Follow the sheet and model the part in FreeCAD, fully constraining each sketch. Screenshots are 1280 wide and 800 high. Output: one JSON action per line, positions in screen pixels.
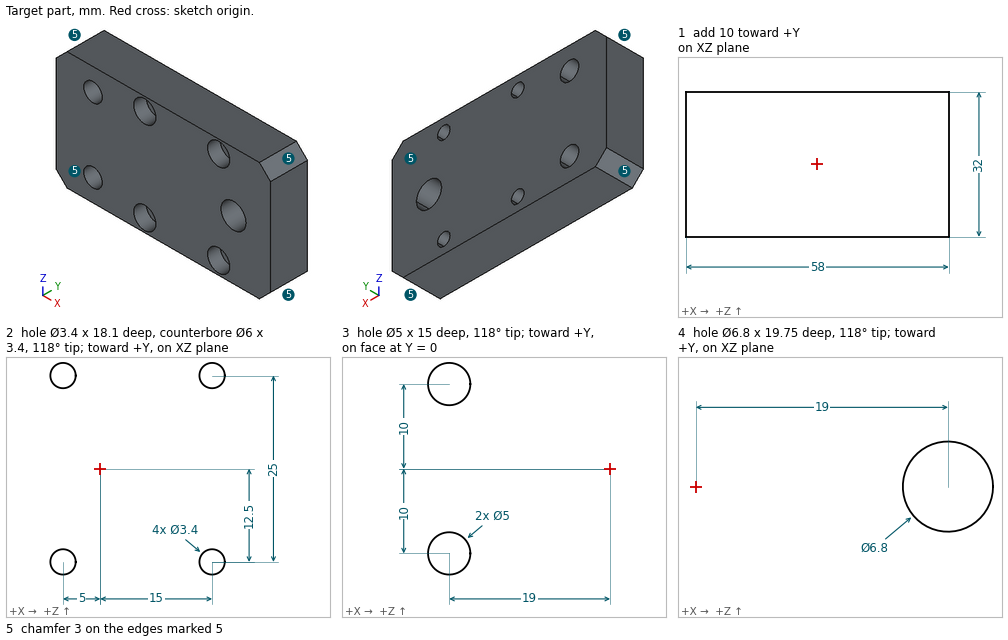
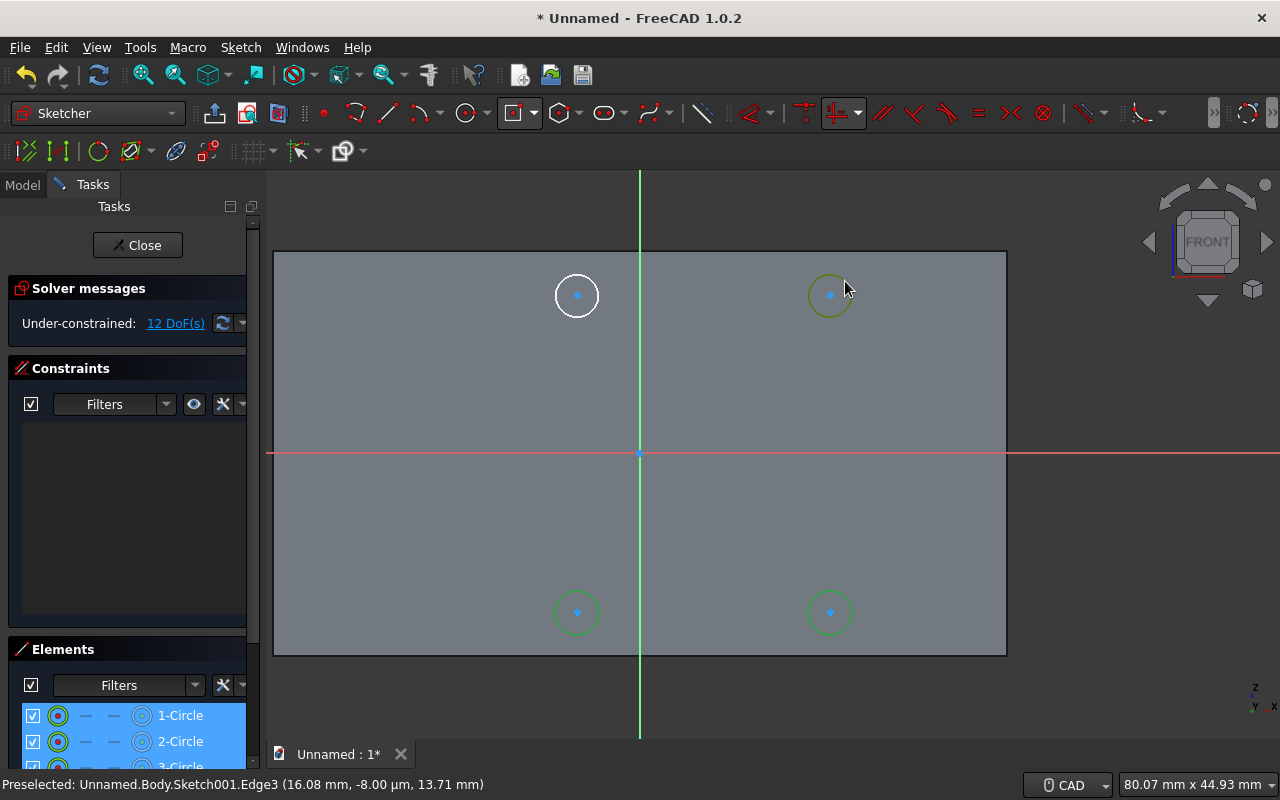
{"action": "left_click", "coordinate": [592, 281]}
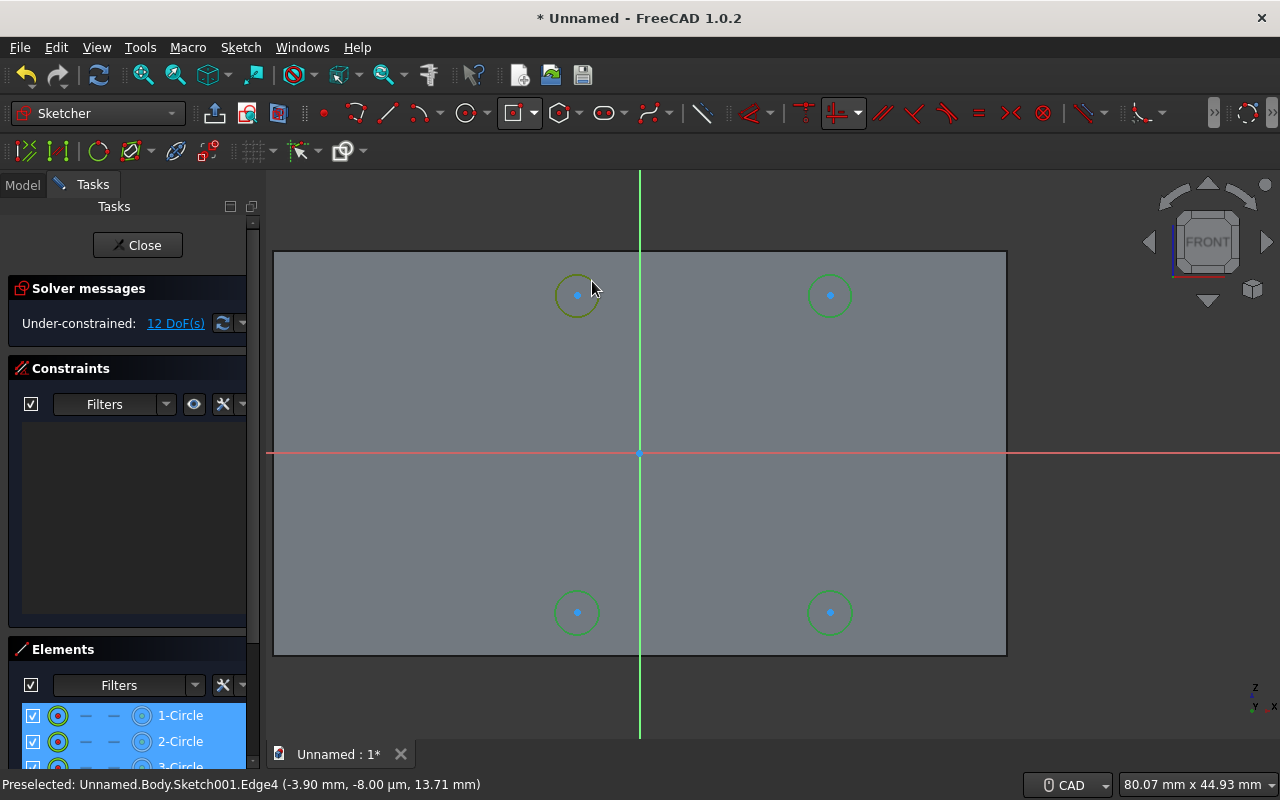
{"action": "left_click", "coordinate": [980, 114]}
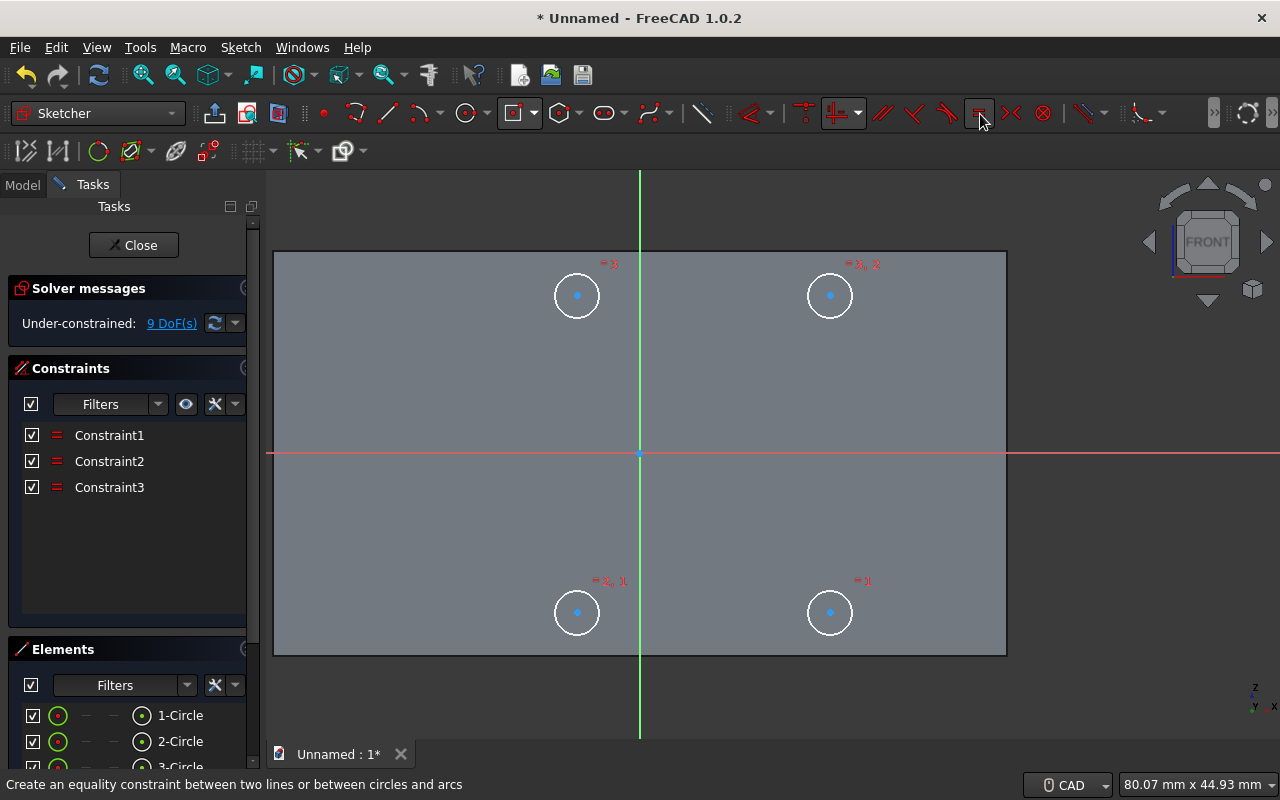
{"action": "left_click", "coordinate": [830, 613]}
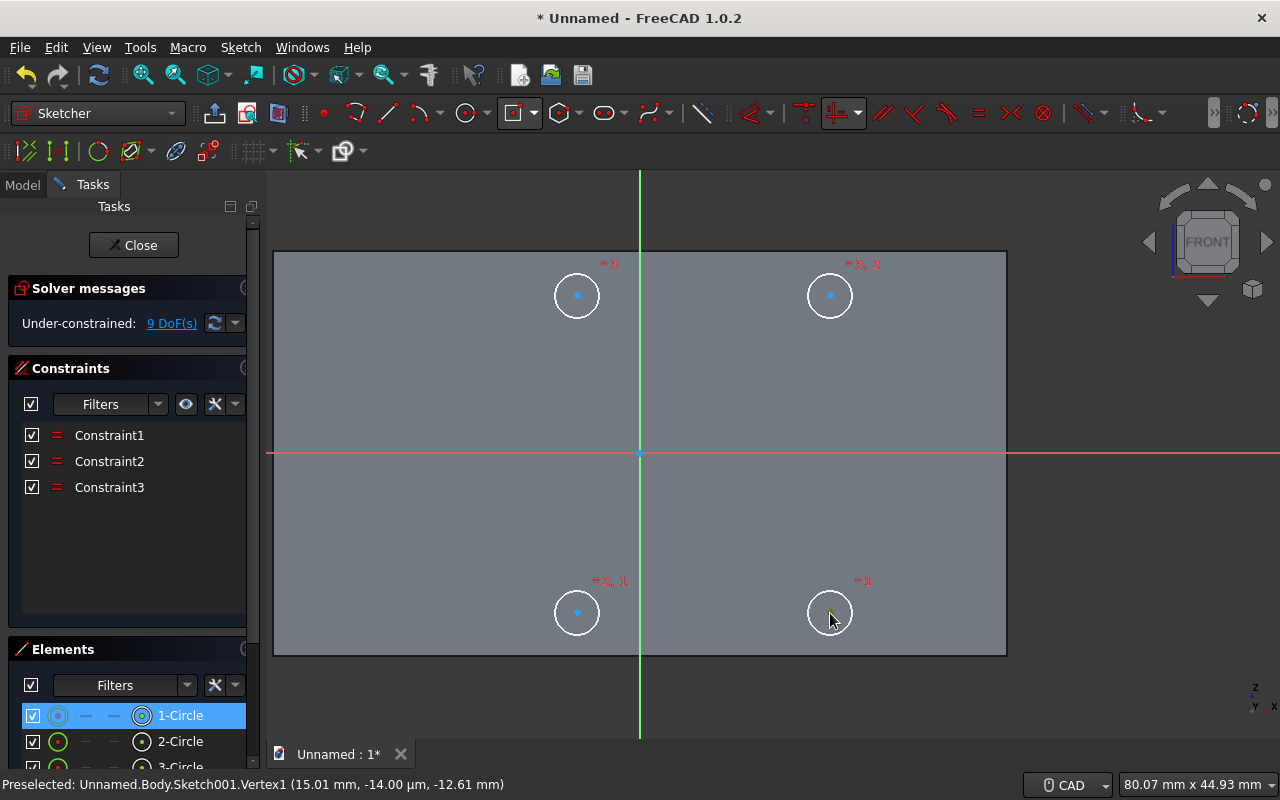
{"action": "left_click", "coordinate": [577, 613]}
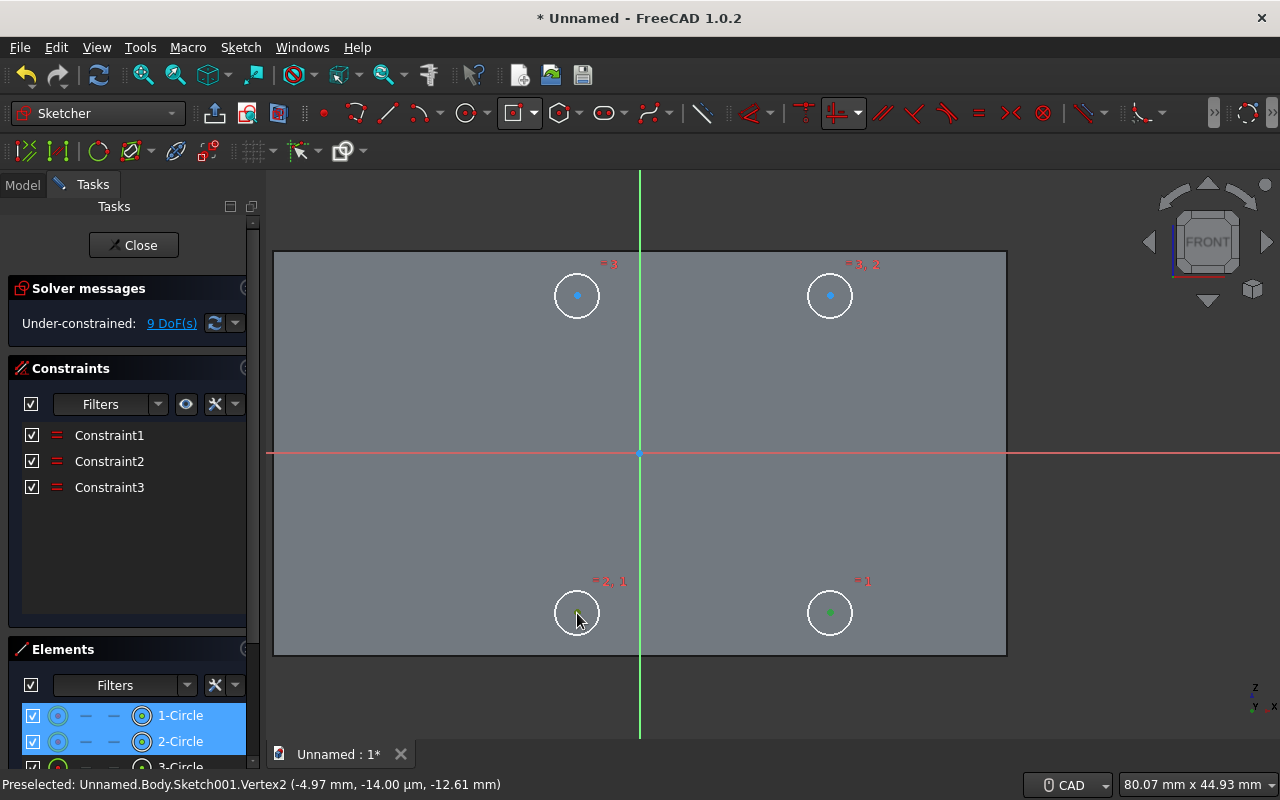
{"action": "key", "text": "h"}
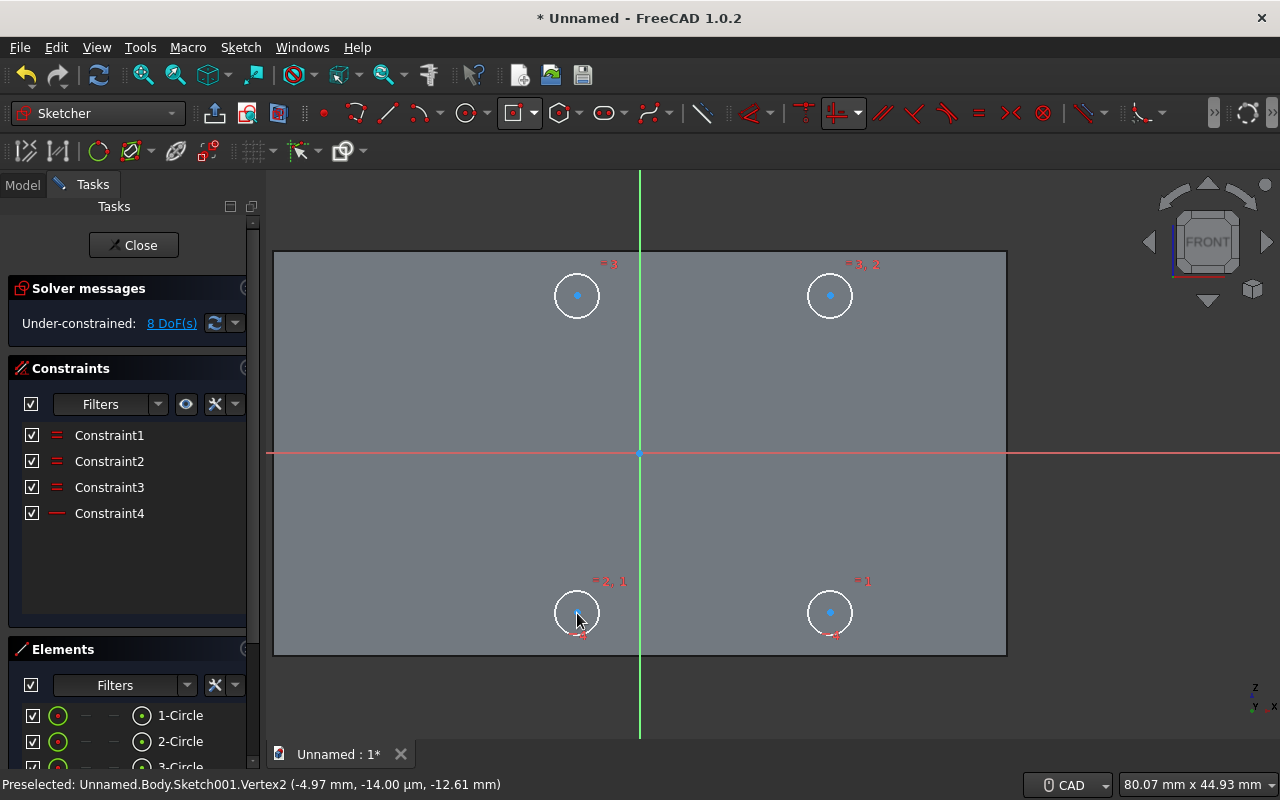
{"action": "left_click", "coordinate": [830, 613]}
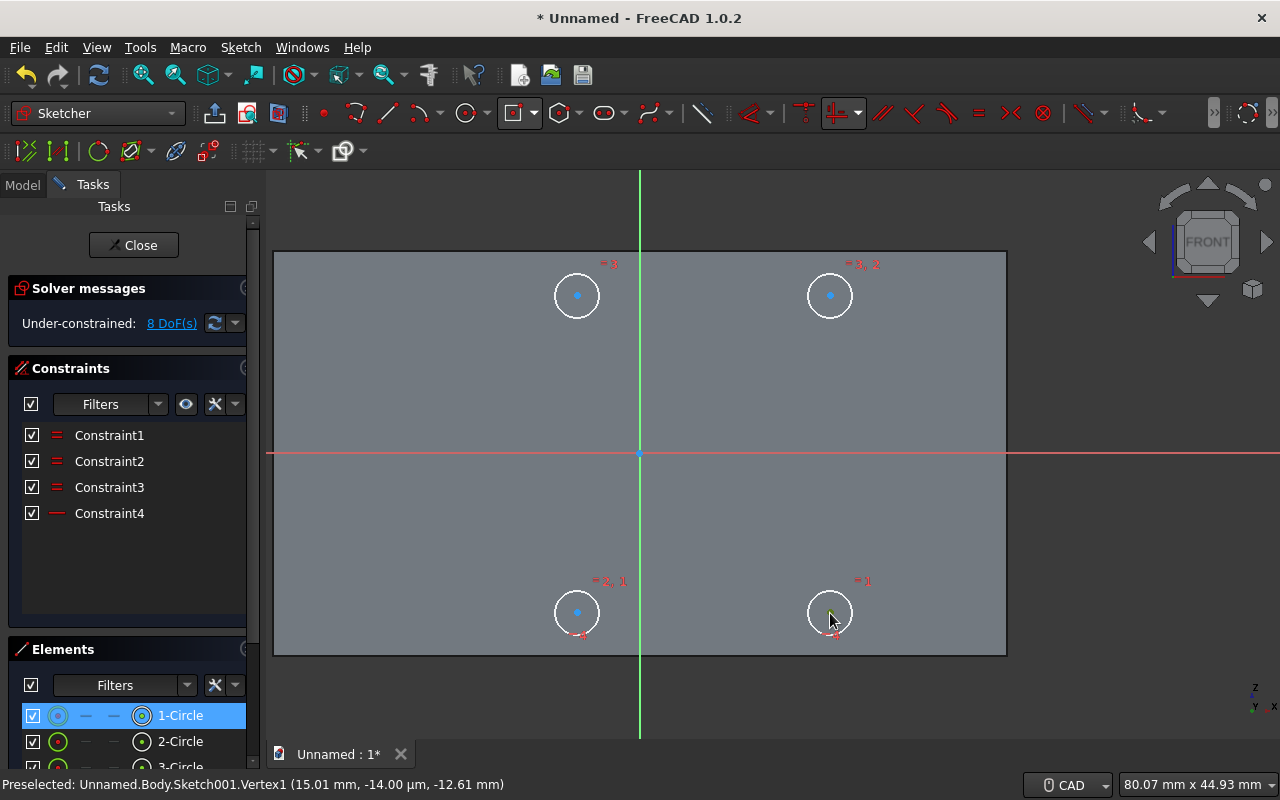
{"action": "left_click", "coordinate": [830, 296]}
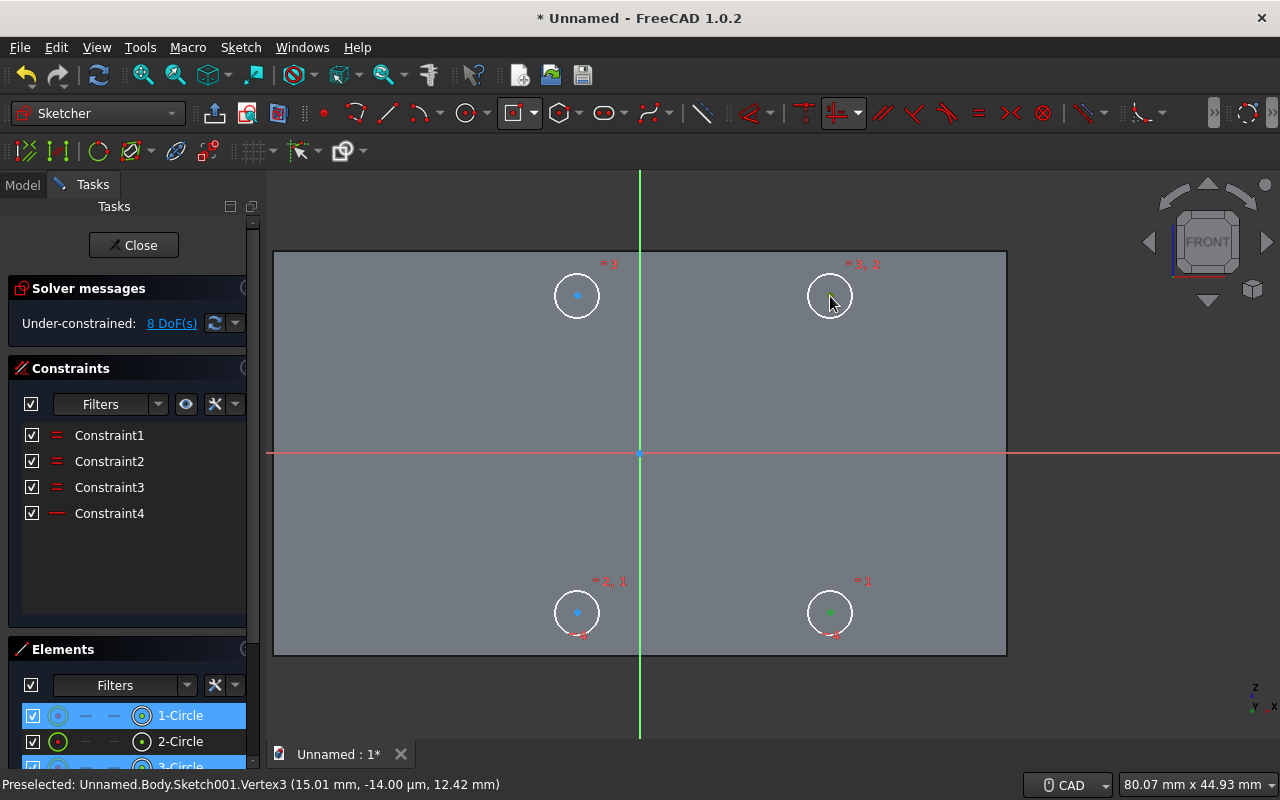
{"action": "left_click", "coordinate": [860, 114]}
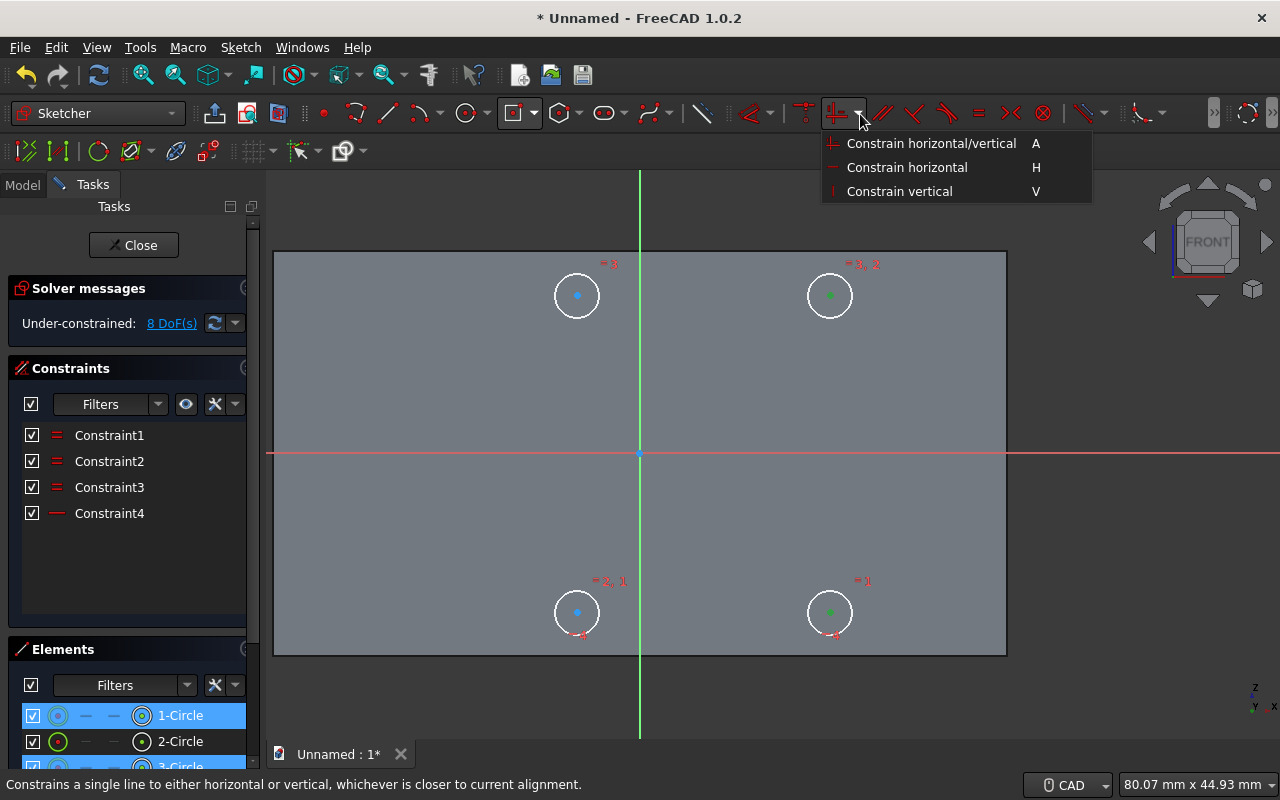
{"action": "left_click", "coordinate": [957, 191]}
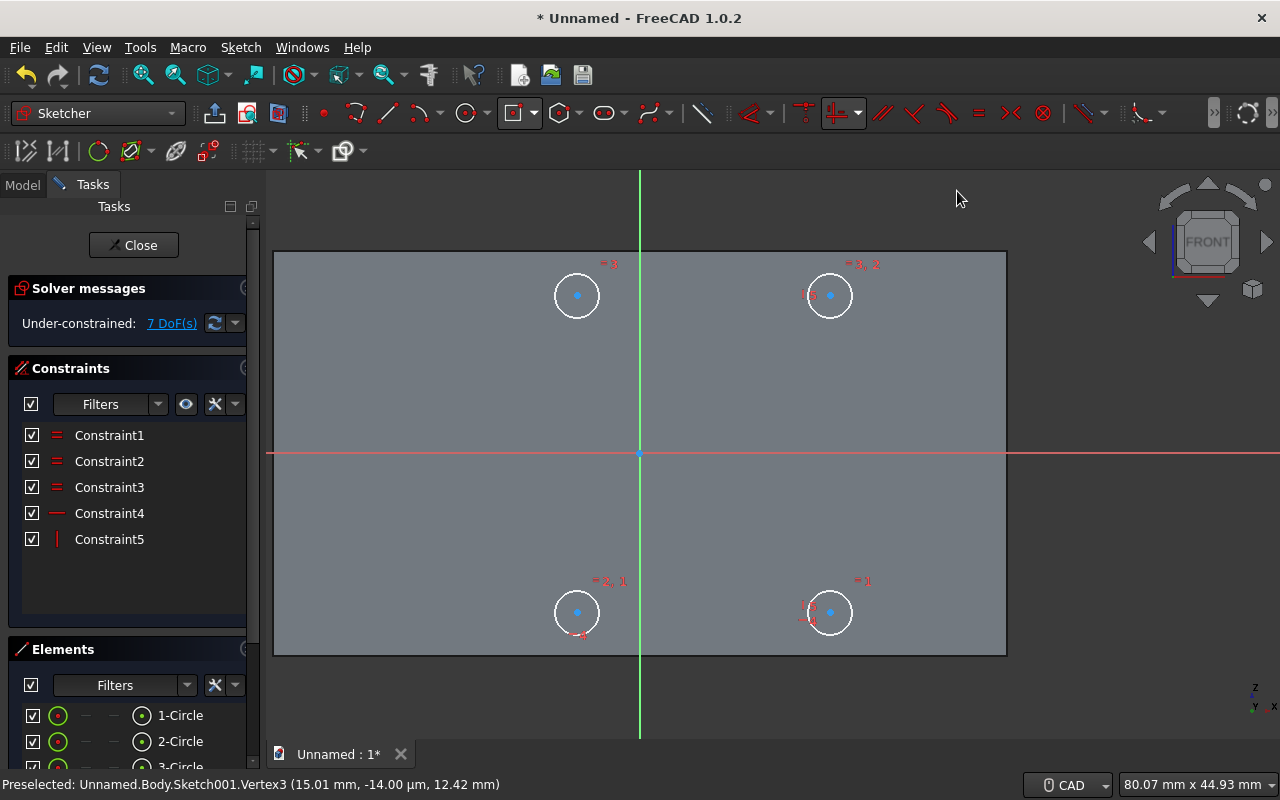
{"action": "left_click", "coordinate": [577, 613]}